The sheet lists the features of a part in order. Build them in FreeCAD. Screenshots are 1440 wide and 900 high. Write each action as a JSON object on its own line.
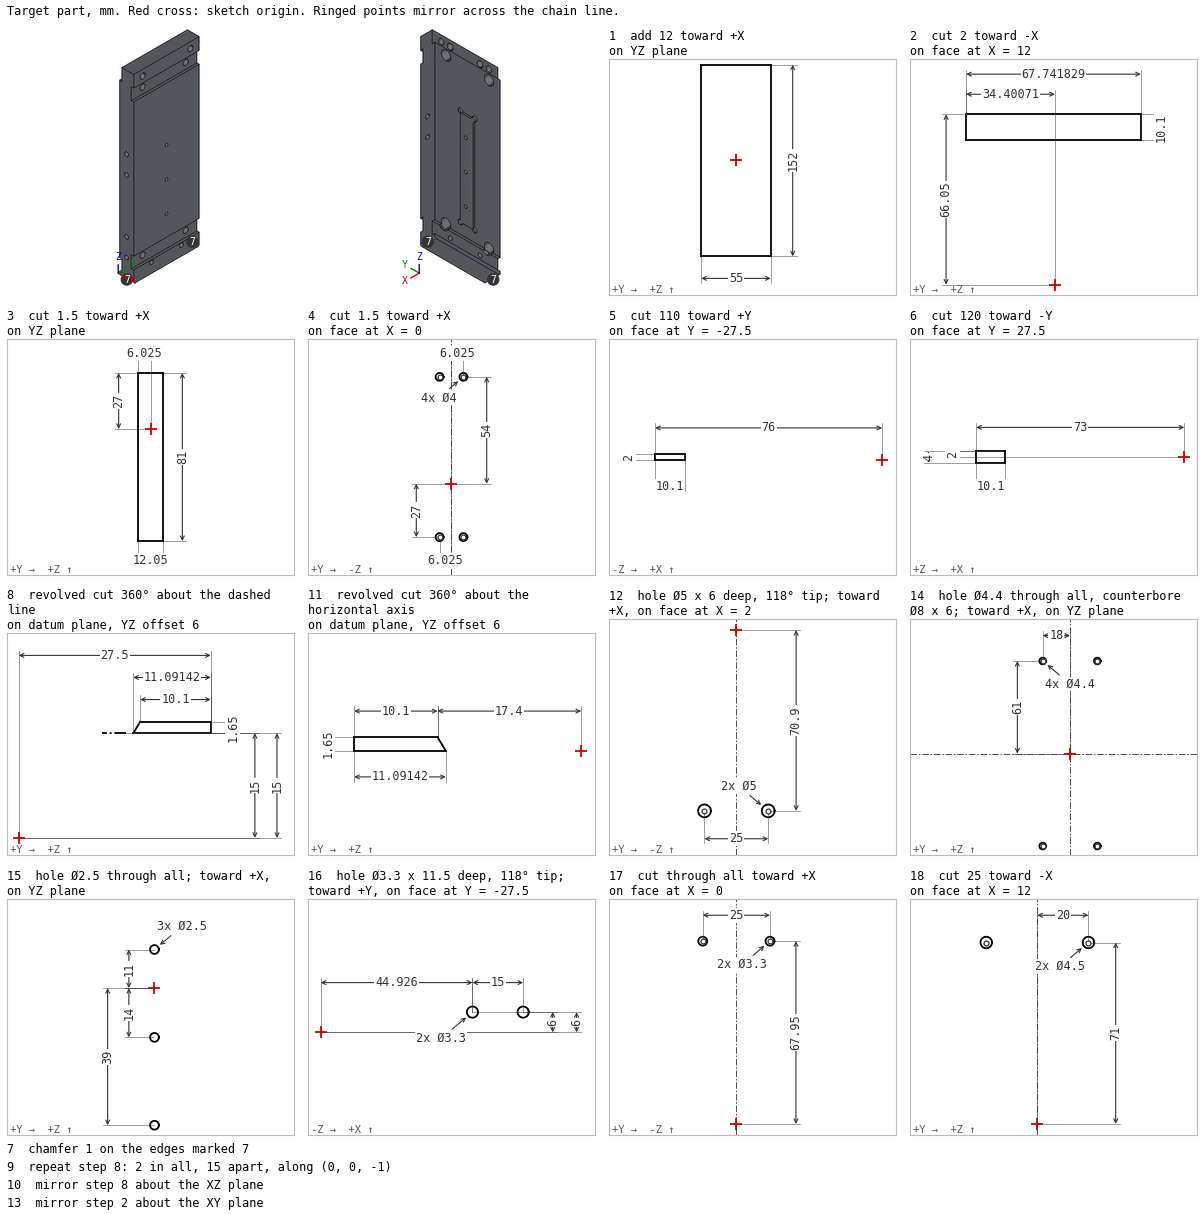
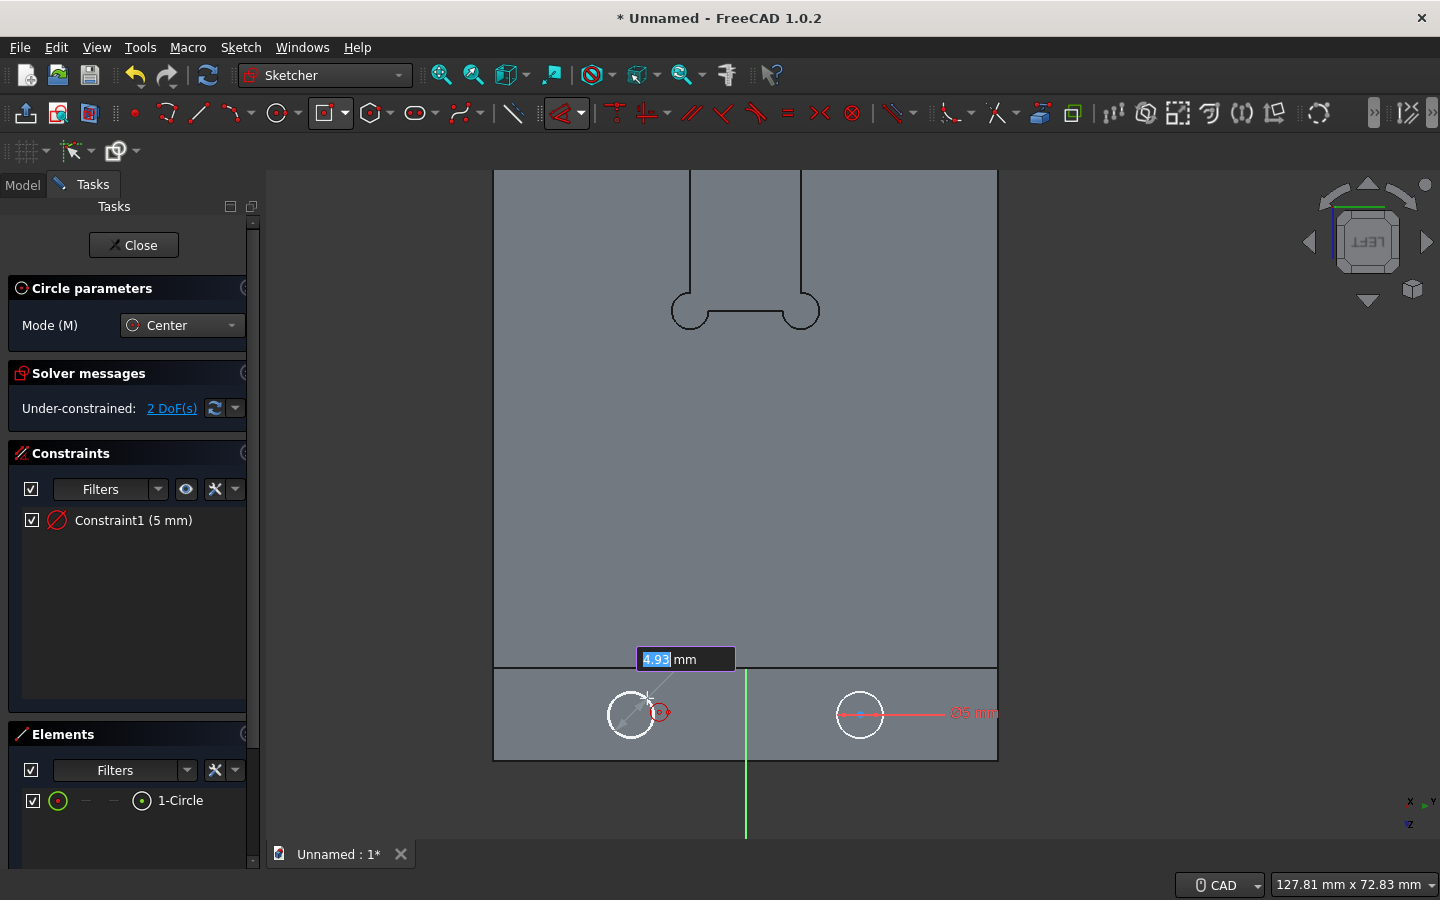
{"action": "type", "text": "5"}
{"action": "key", "text": "Return"}
{"action": "key", "text": "Escape"}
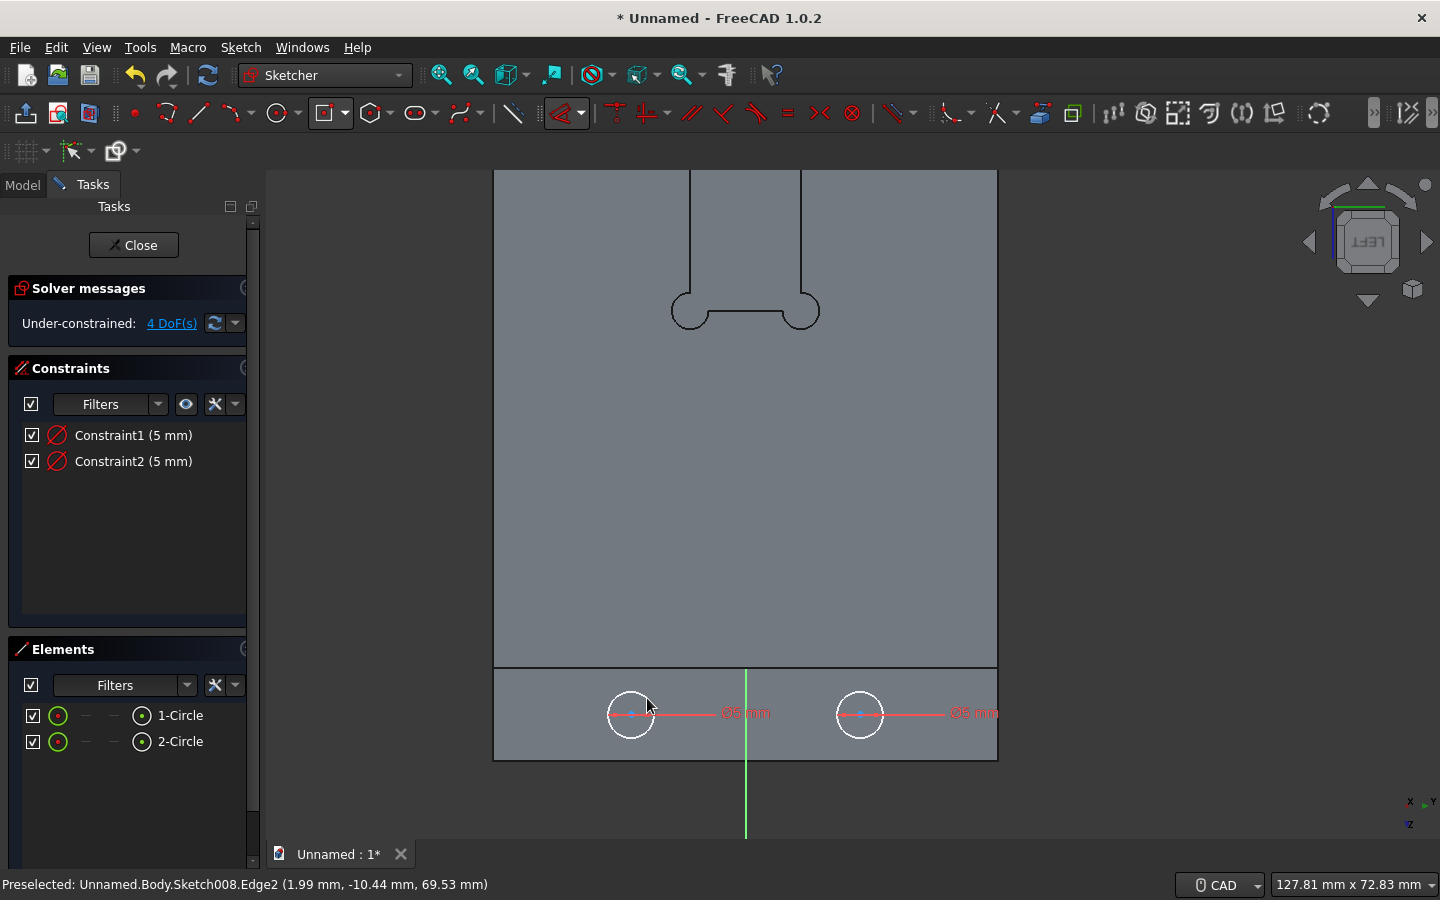
{"action": "left_click", "coordinate": [860, 715]}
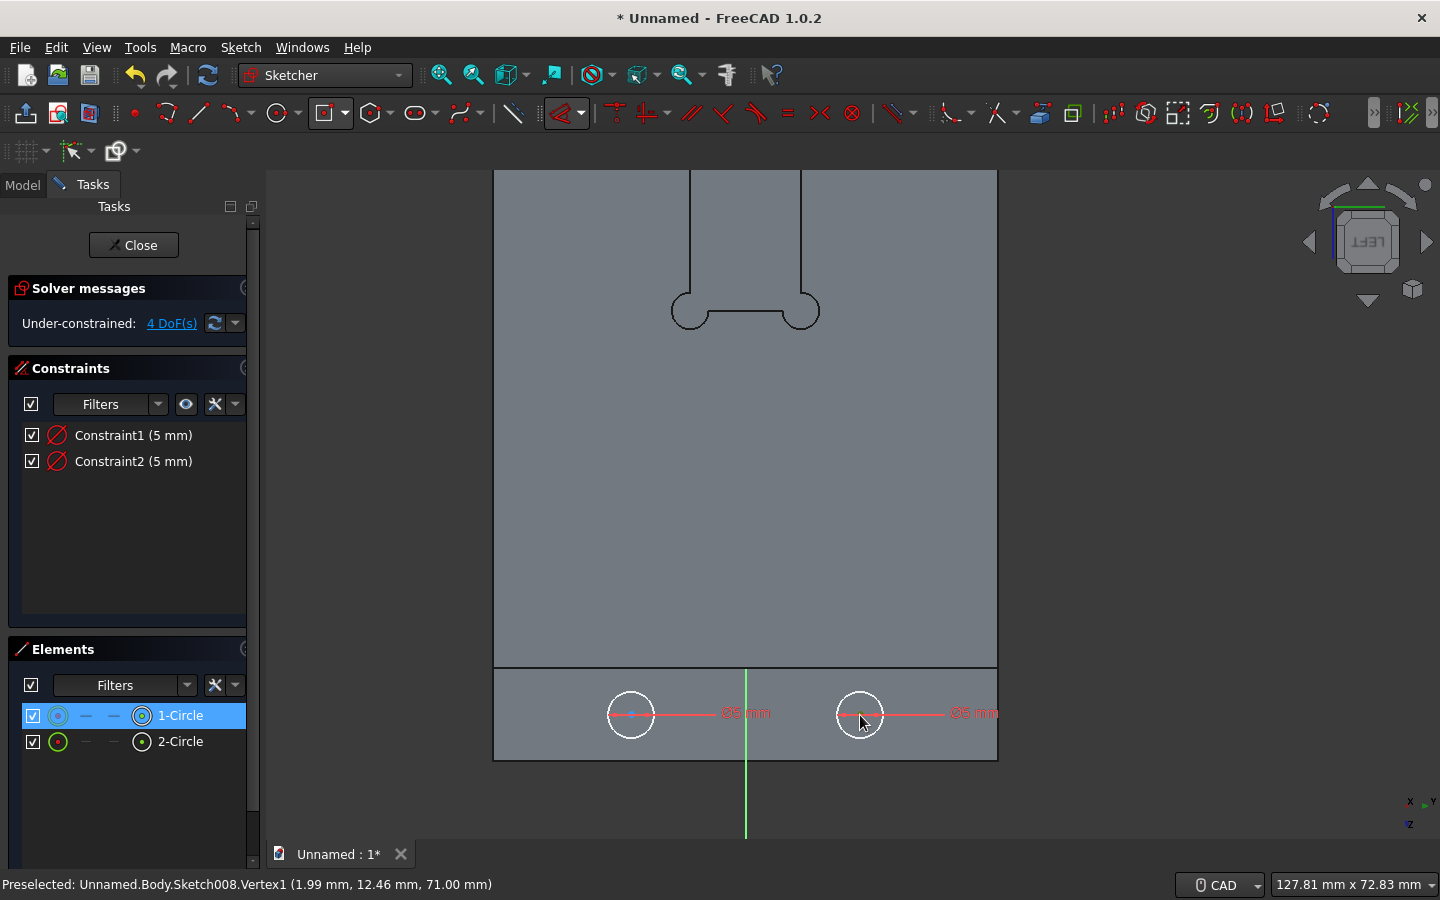
{"action": "left_click", "coordinate": [631, 715]}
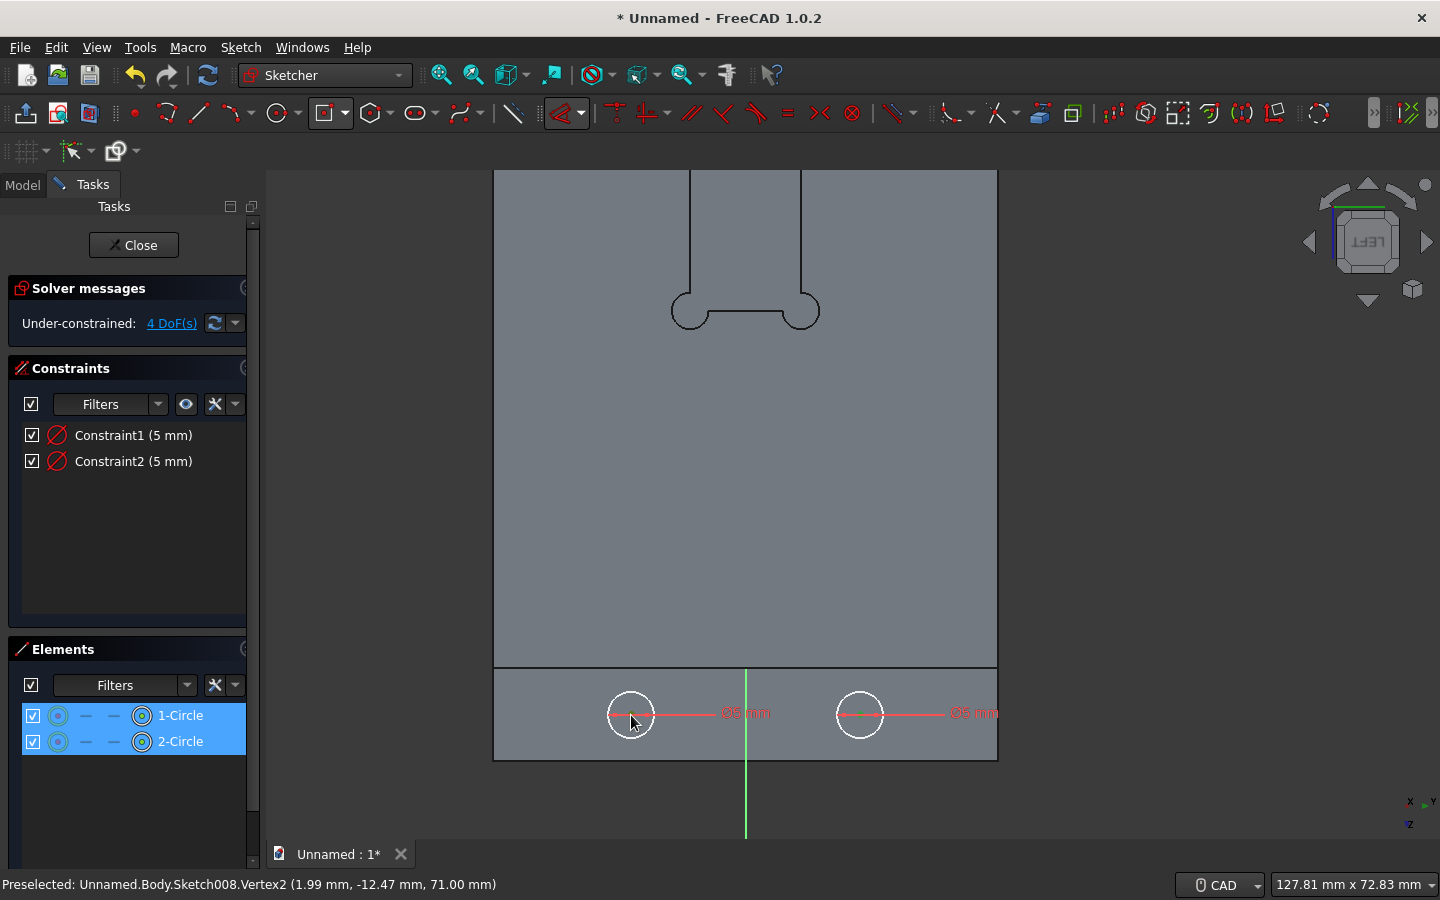
{"action": "left_click", "coordinate": [746, 767]}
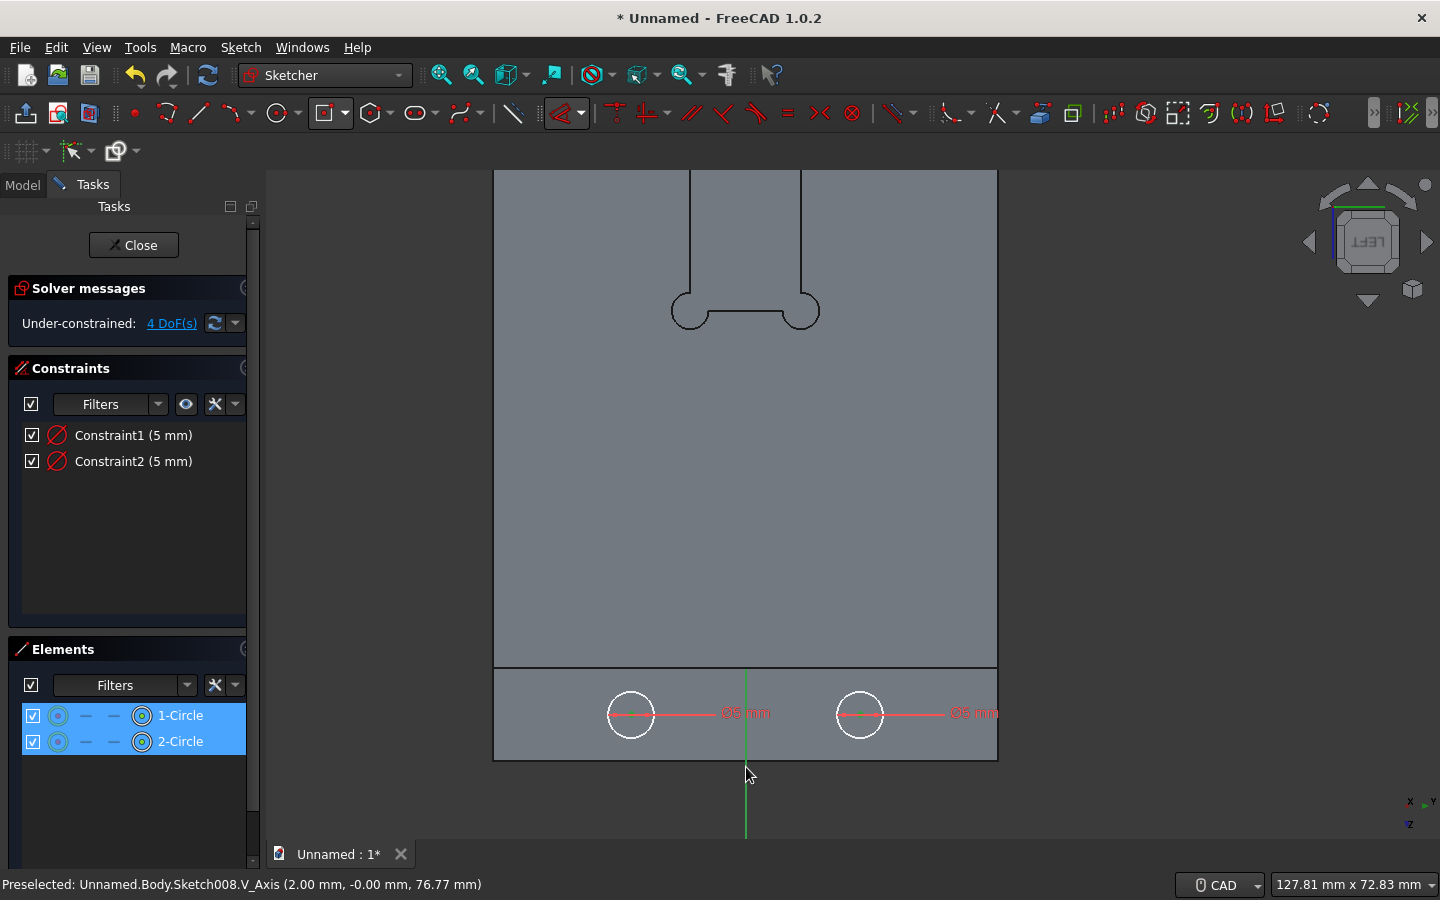
{"action": "key", "text": "s"}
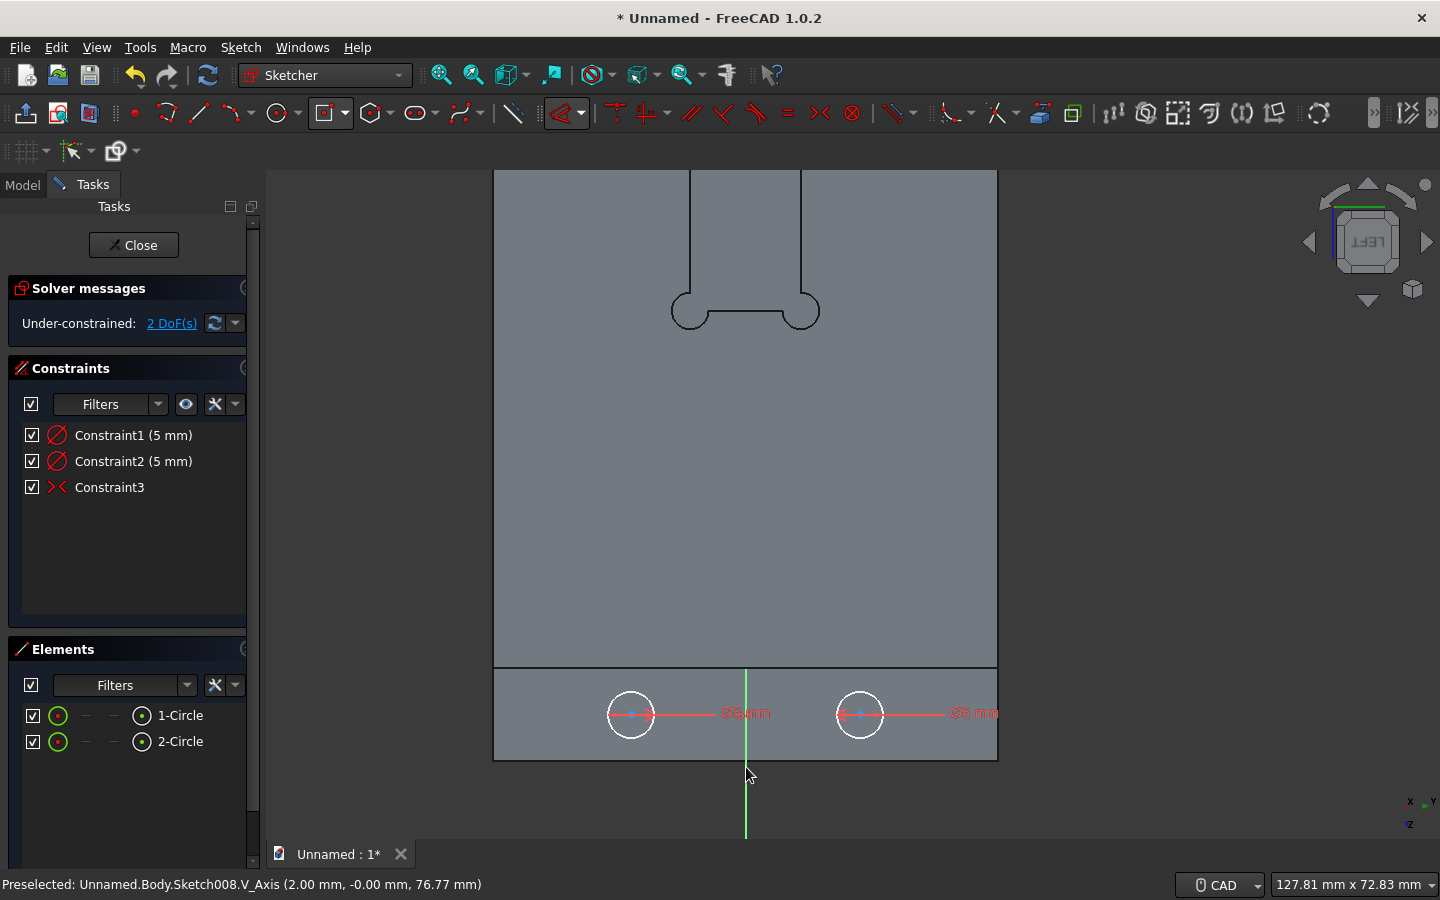
{"action": "left_click", "coordinate": [860, 715]}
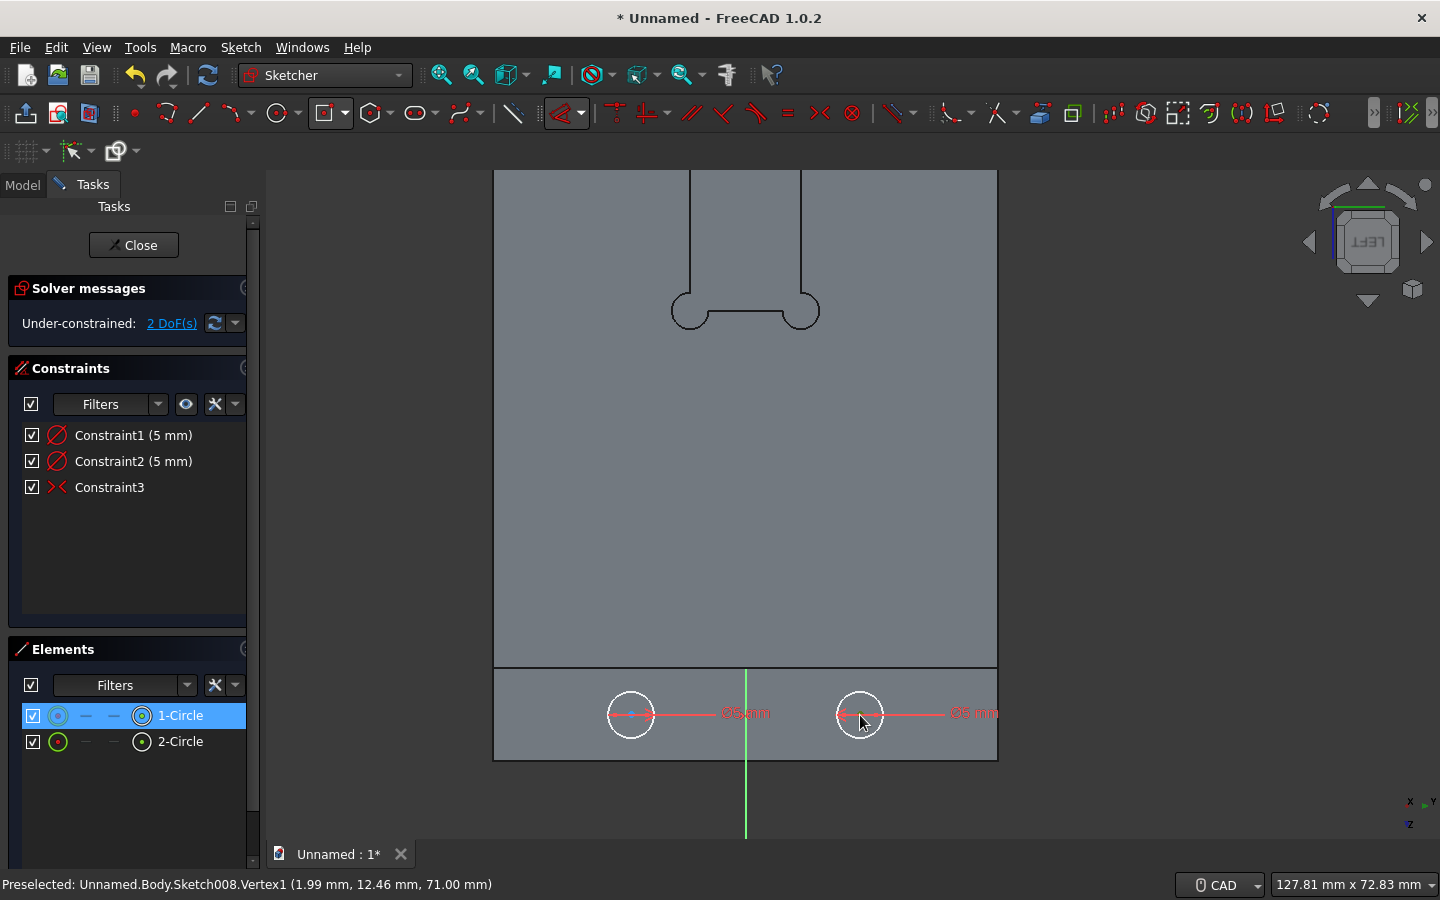
{"action": "left_click", "coordinate": [631, 715]}